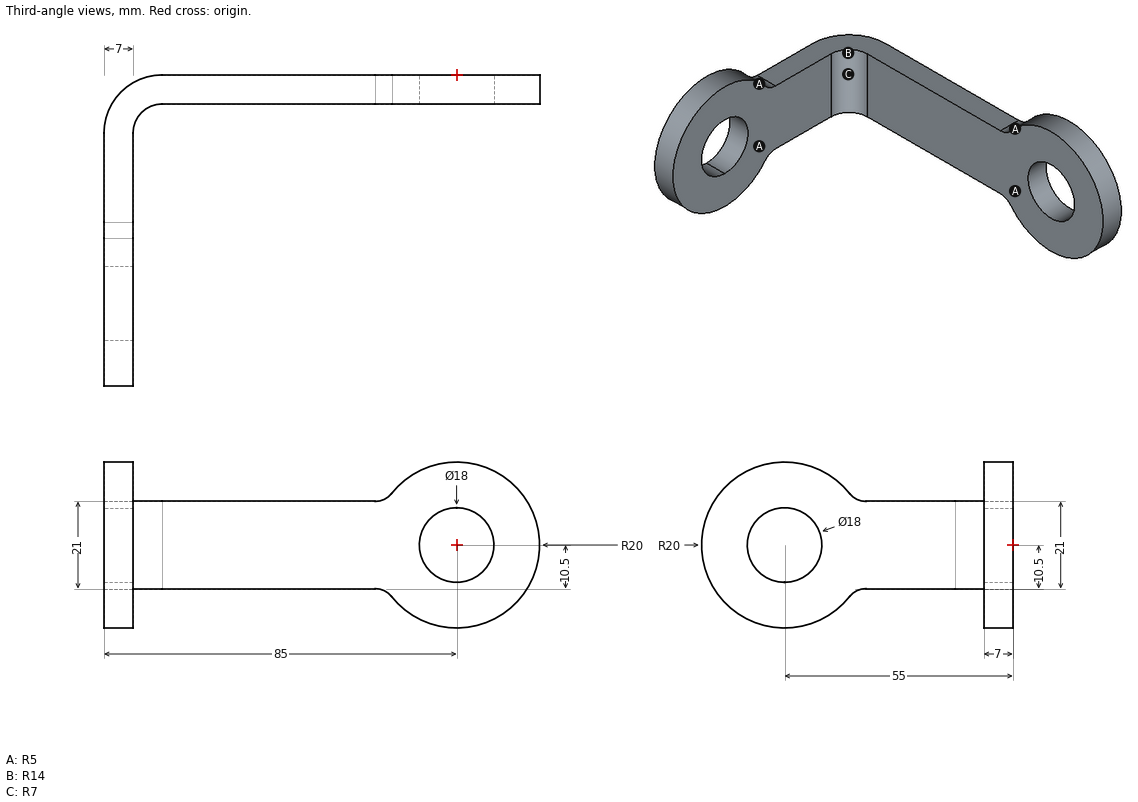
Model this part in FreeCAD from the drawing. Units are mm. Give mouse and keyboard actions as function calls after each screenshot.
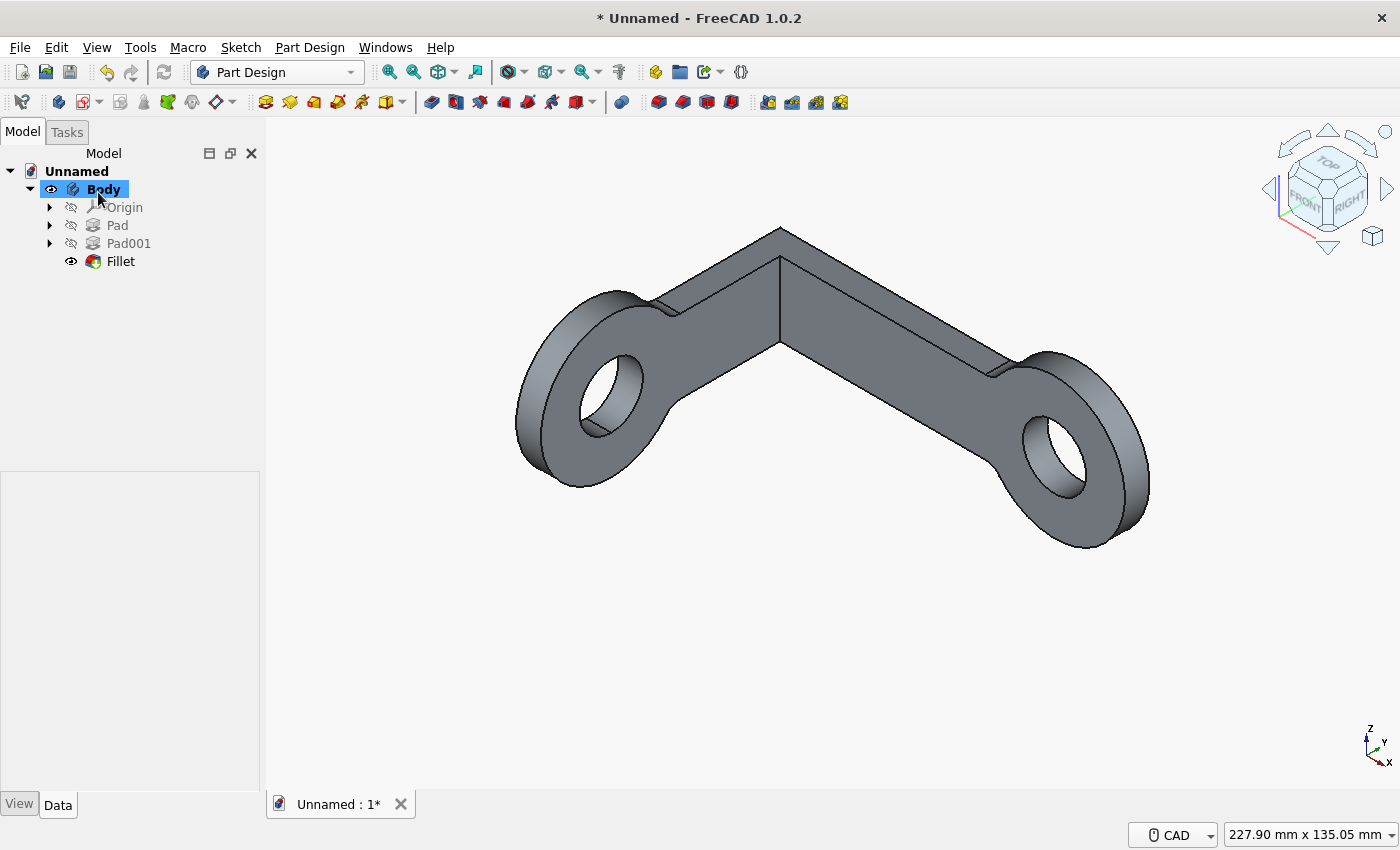
key(2)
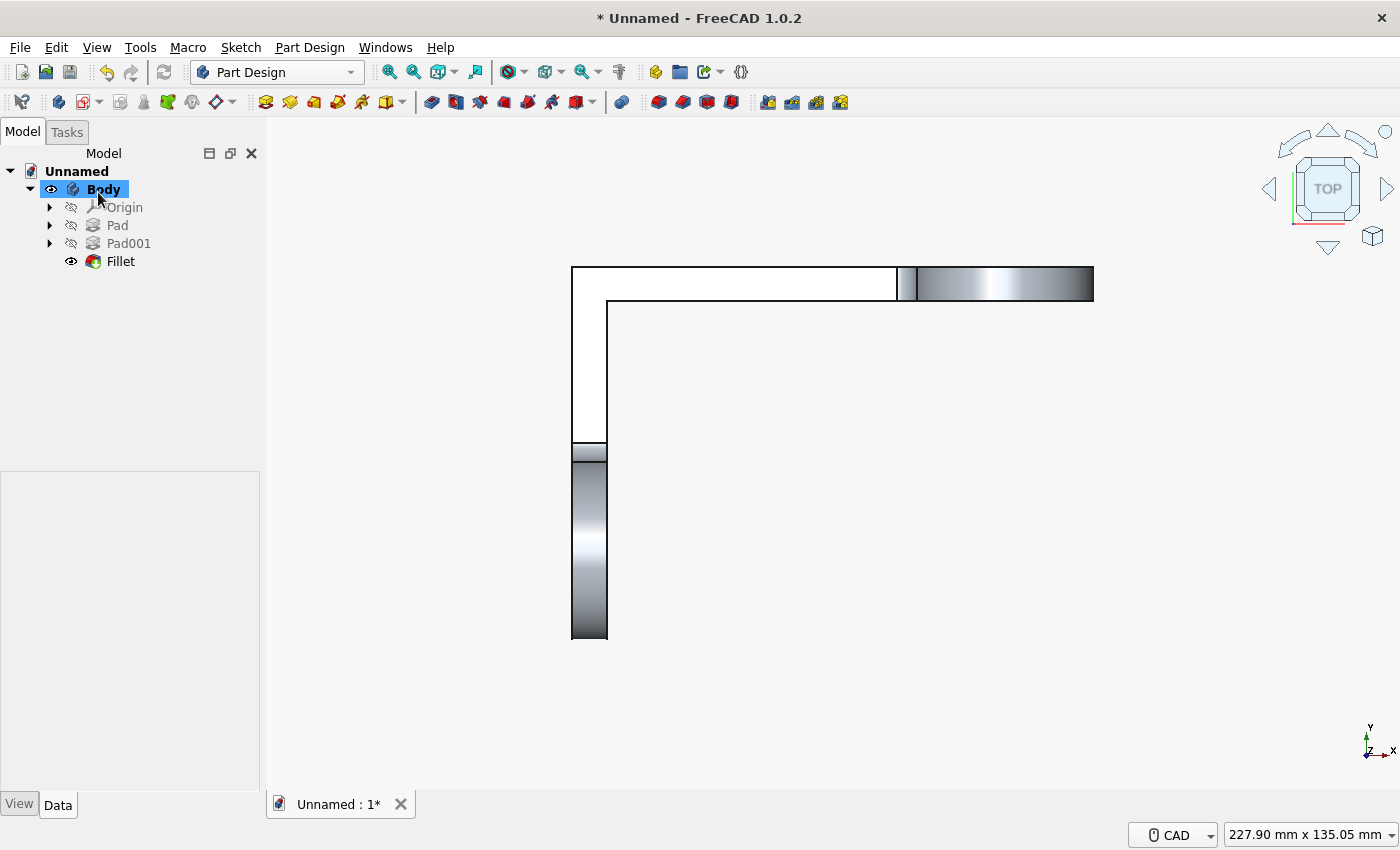
key(1)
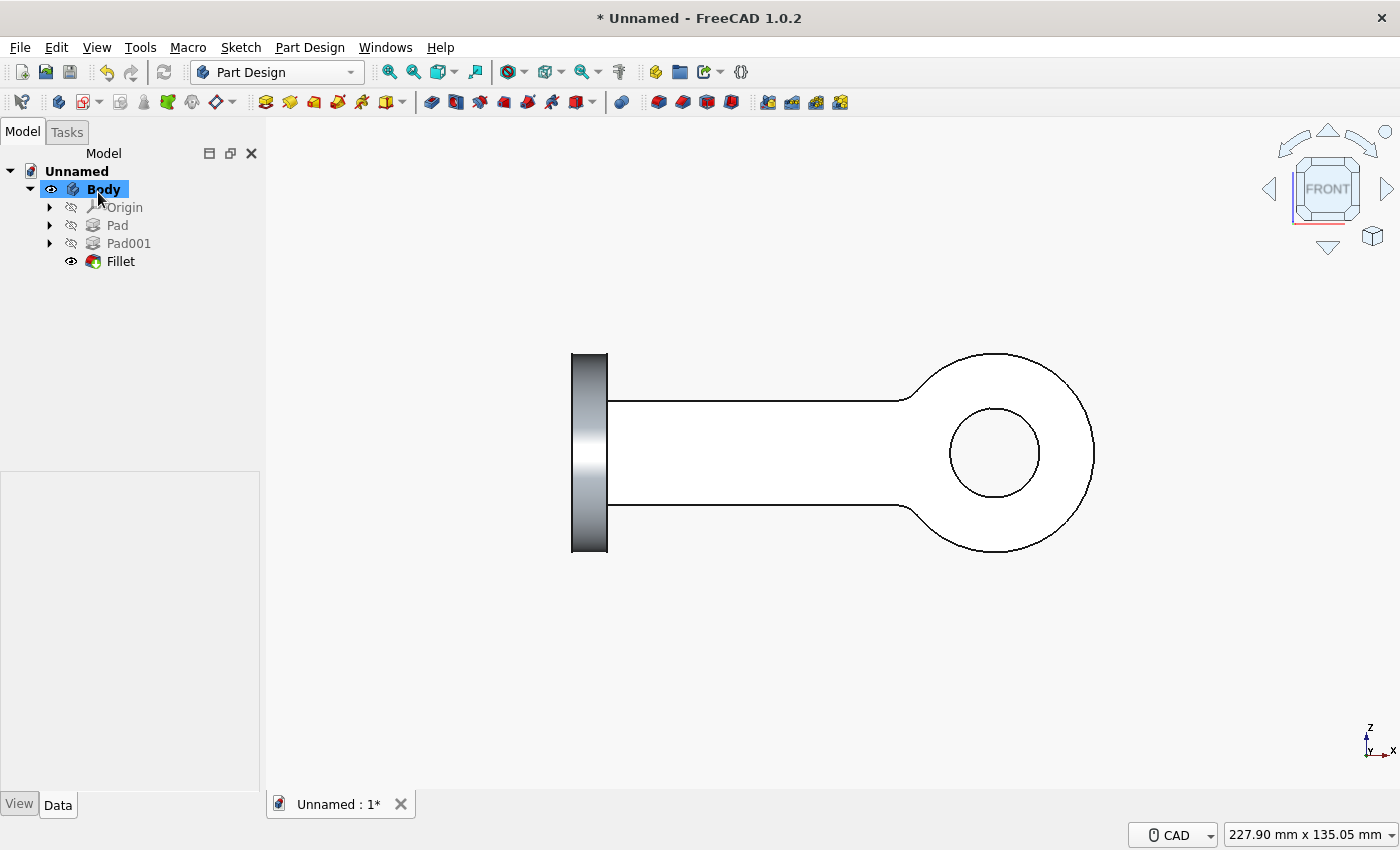
key(3)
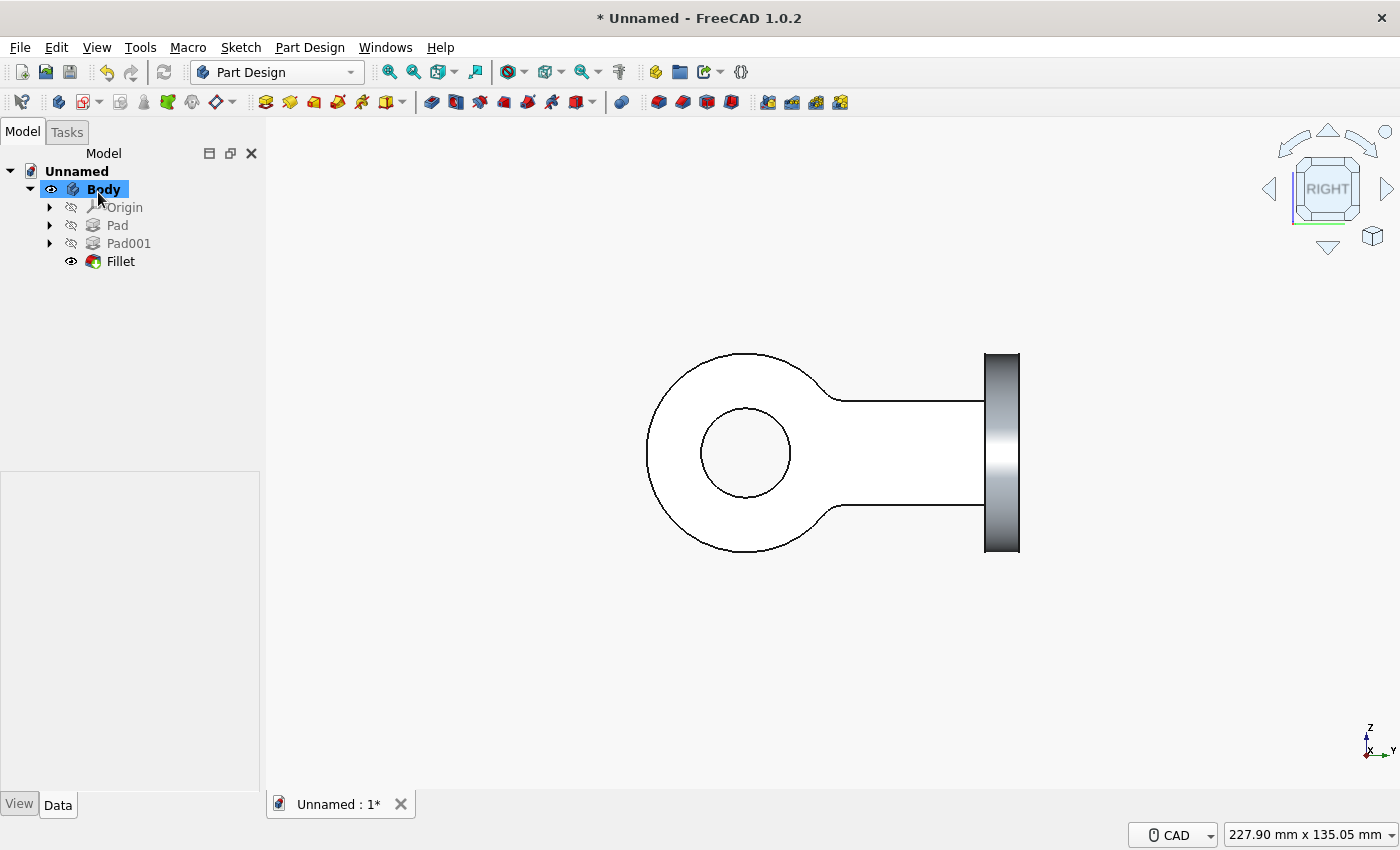
click(390, 72)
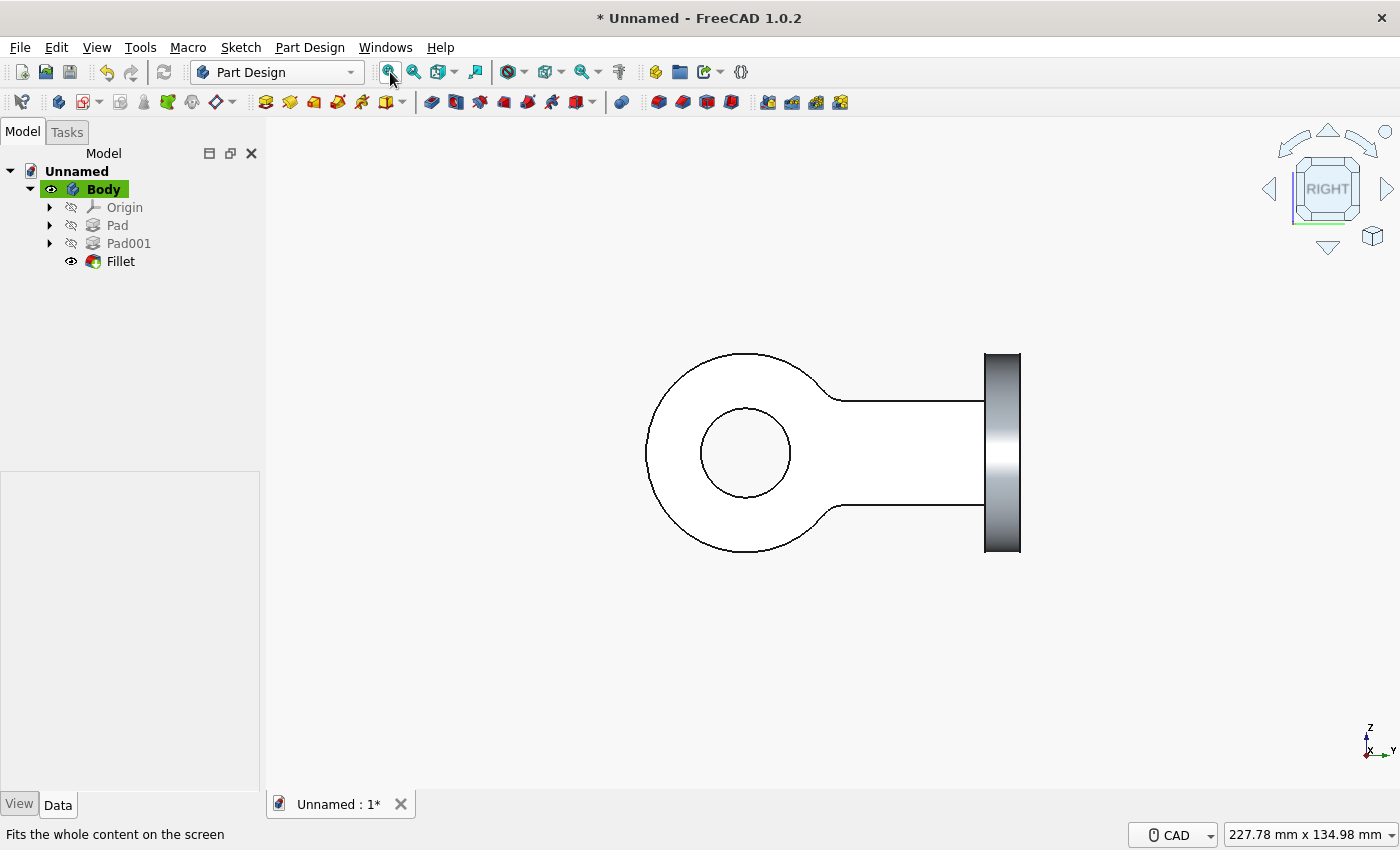
key(5)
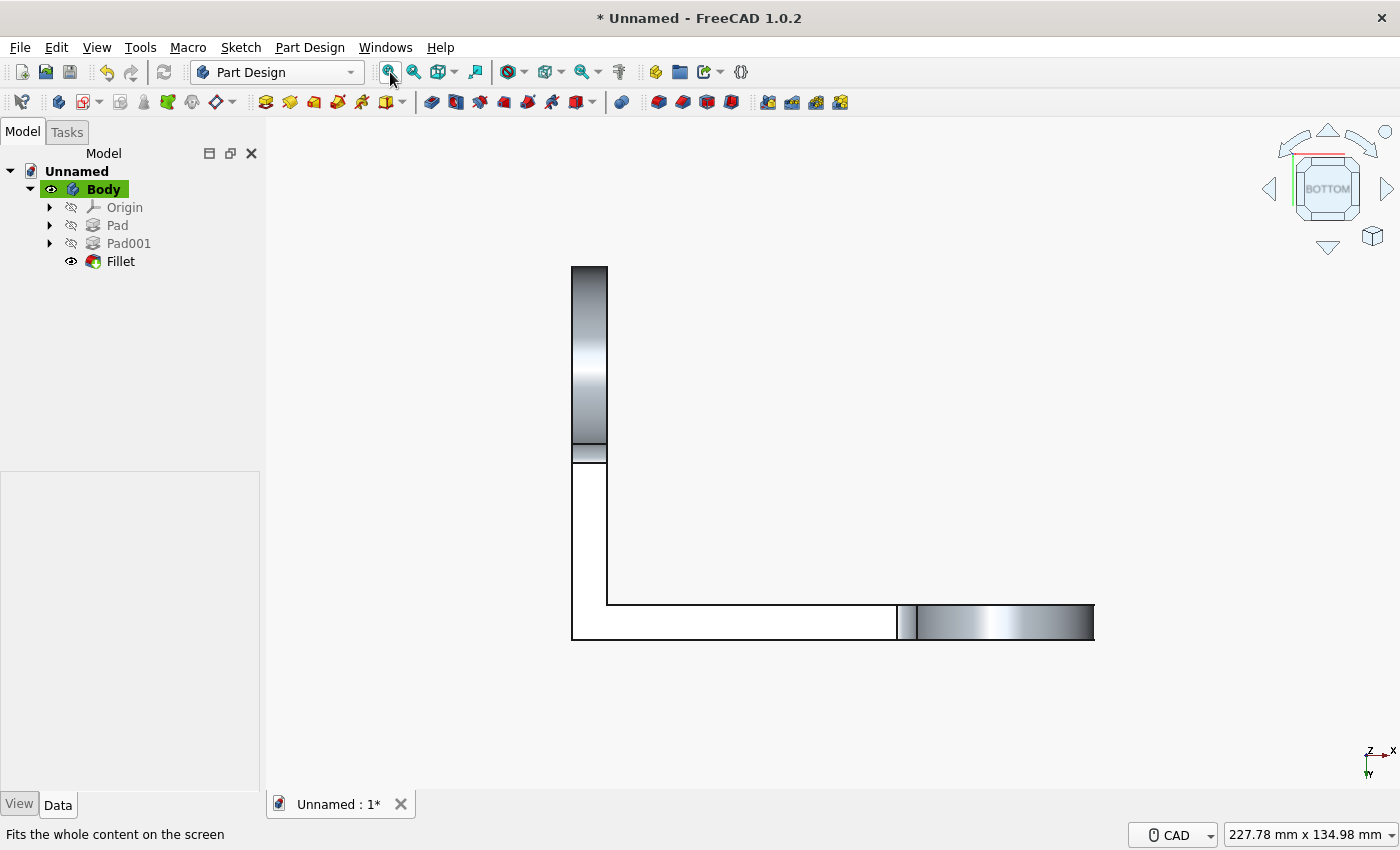
key(4)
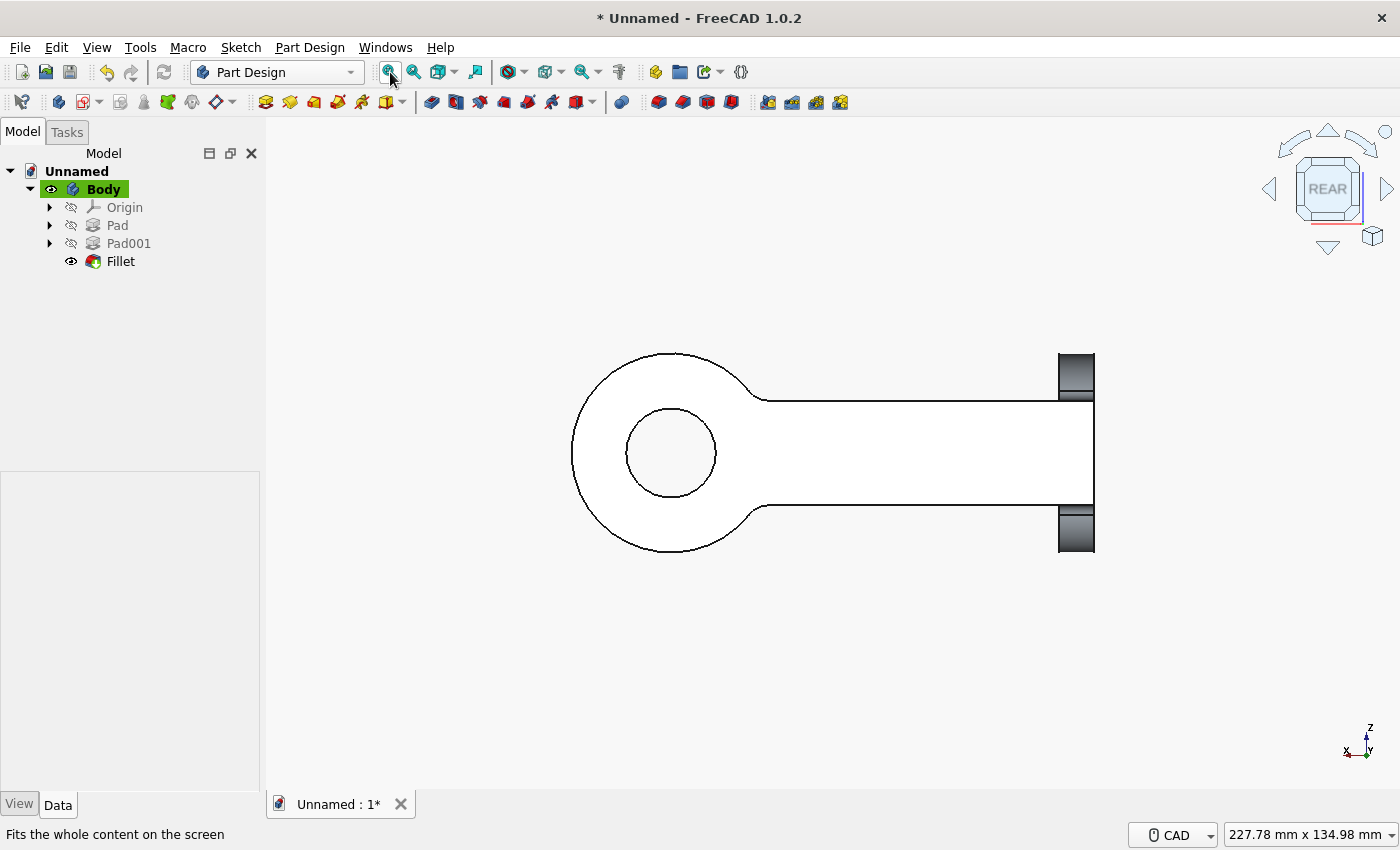
key(6)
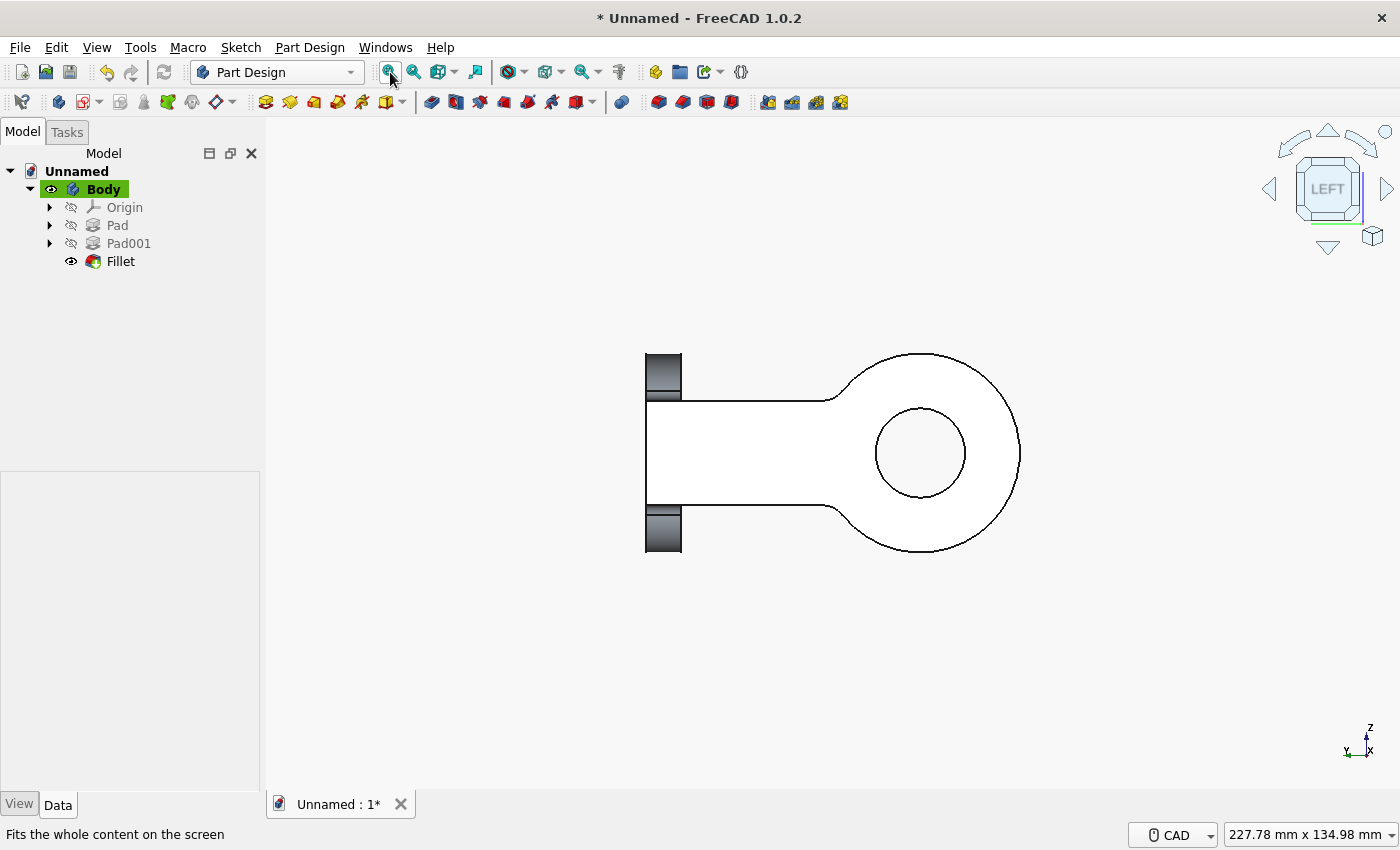
click(390, 72)